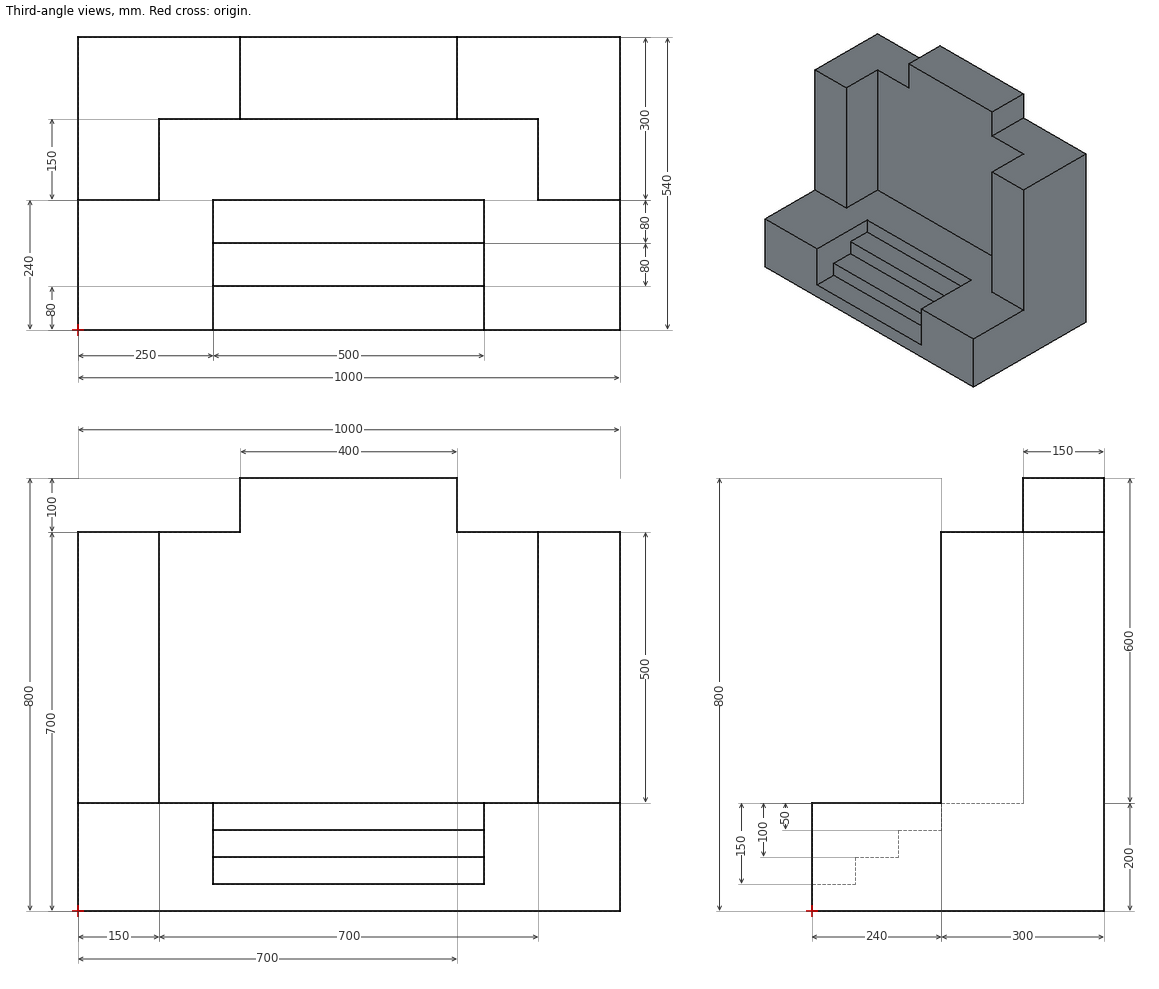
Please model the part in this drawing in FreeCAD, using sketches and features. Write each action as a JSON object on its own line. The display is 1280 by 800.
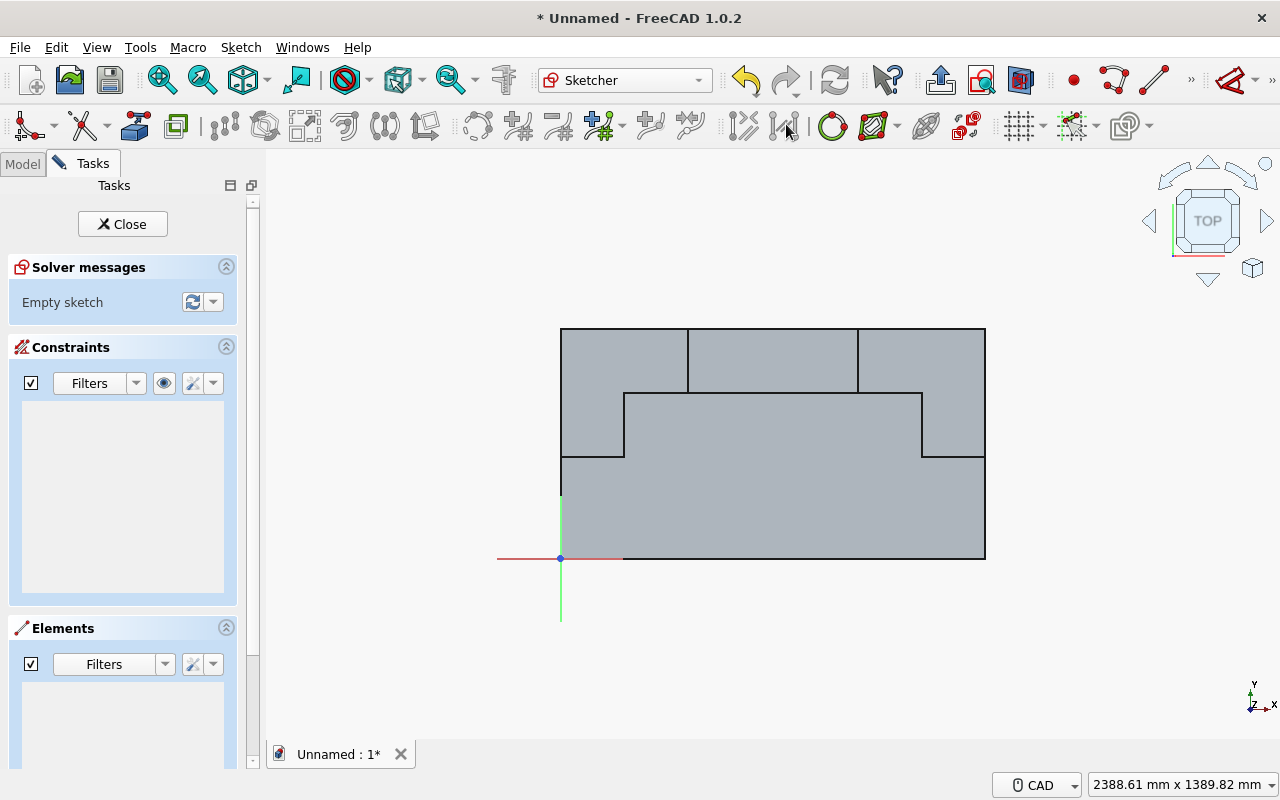
{"action": "scroll", "coordinate": [739, 660], "scroll_direction": "up", "scroll_amount": 3}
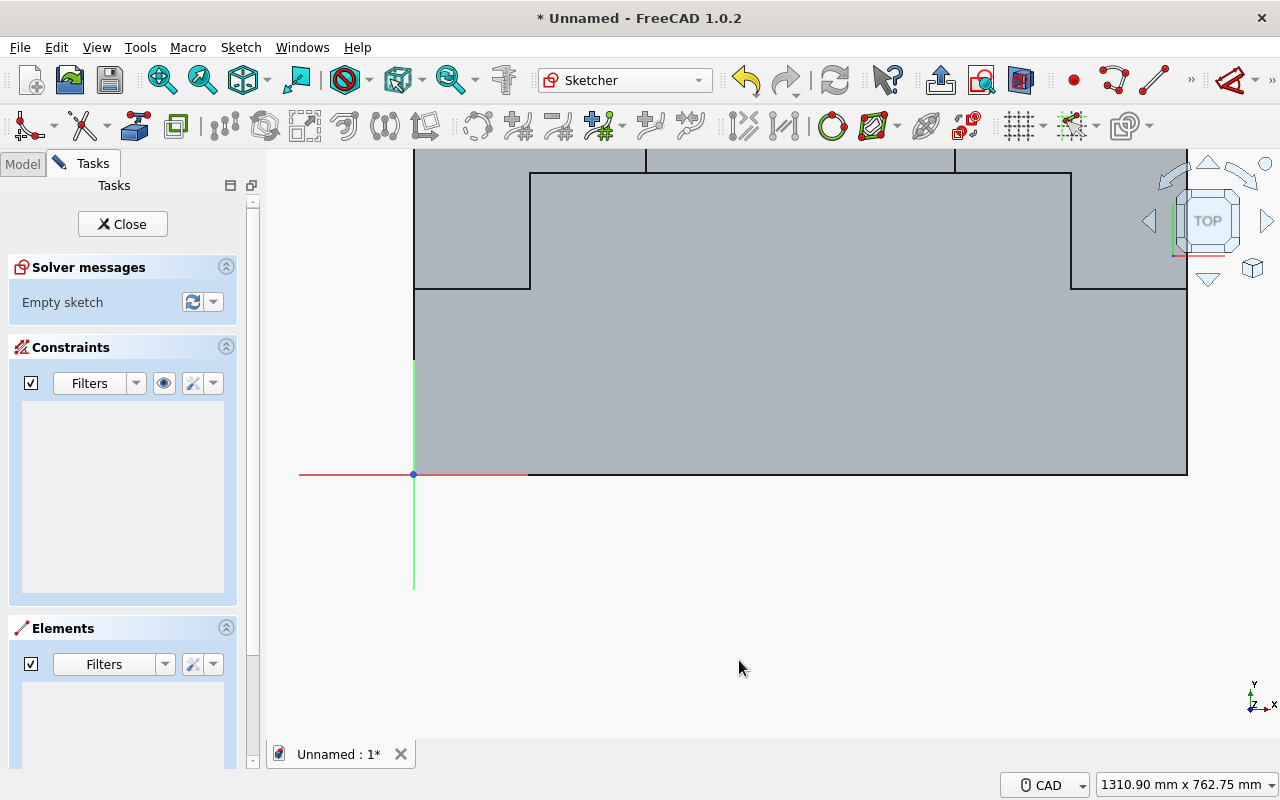
{"action": "key", "text": "g r"}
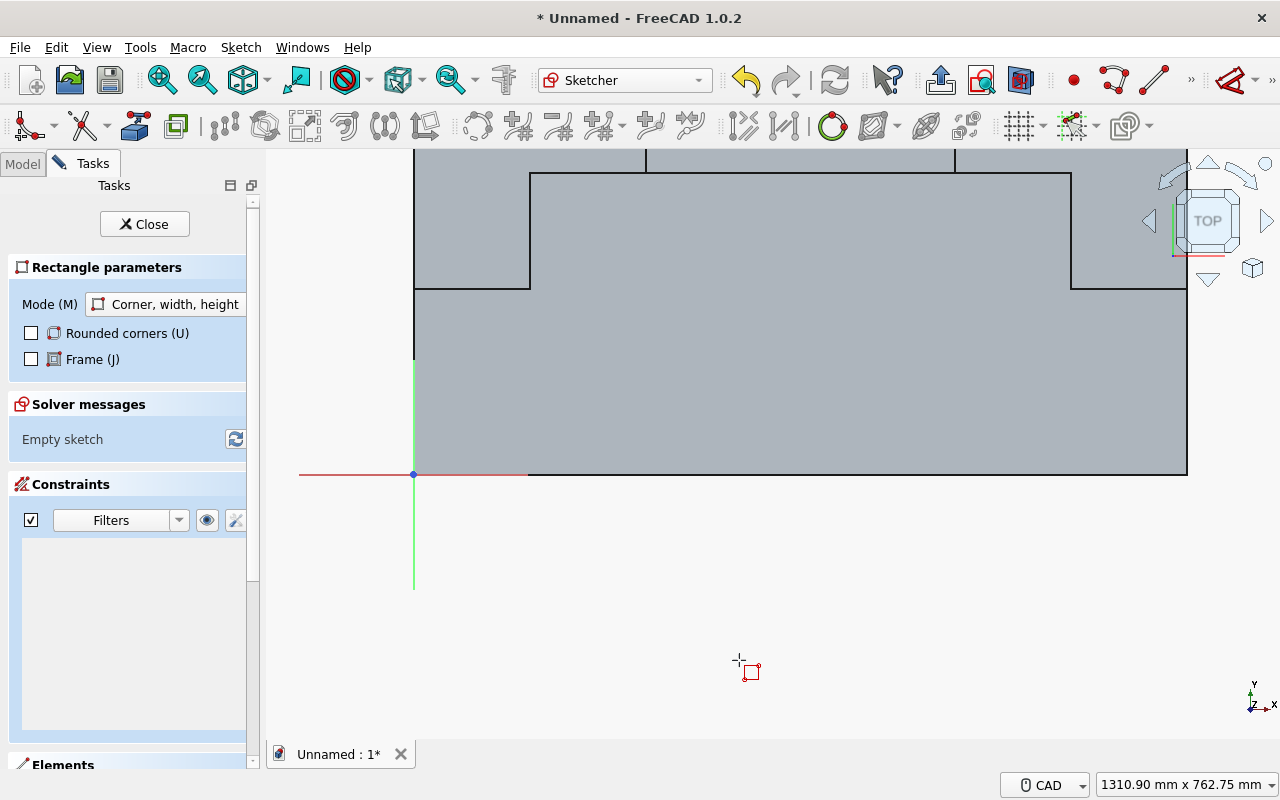
{"action": "left_click", "coordinate": [607, 413]}
{"action": "left_click", "coordinate": [994, 475]}
{"action": "key", "text": "Escape"}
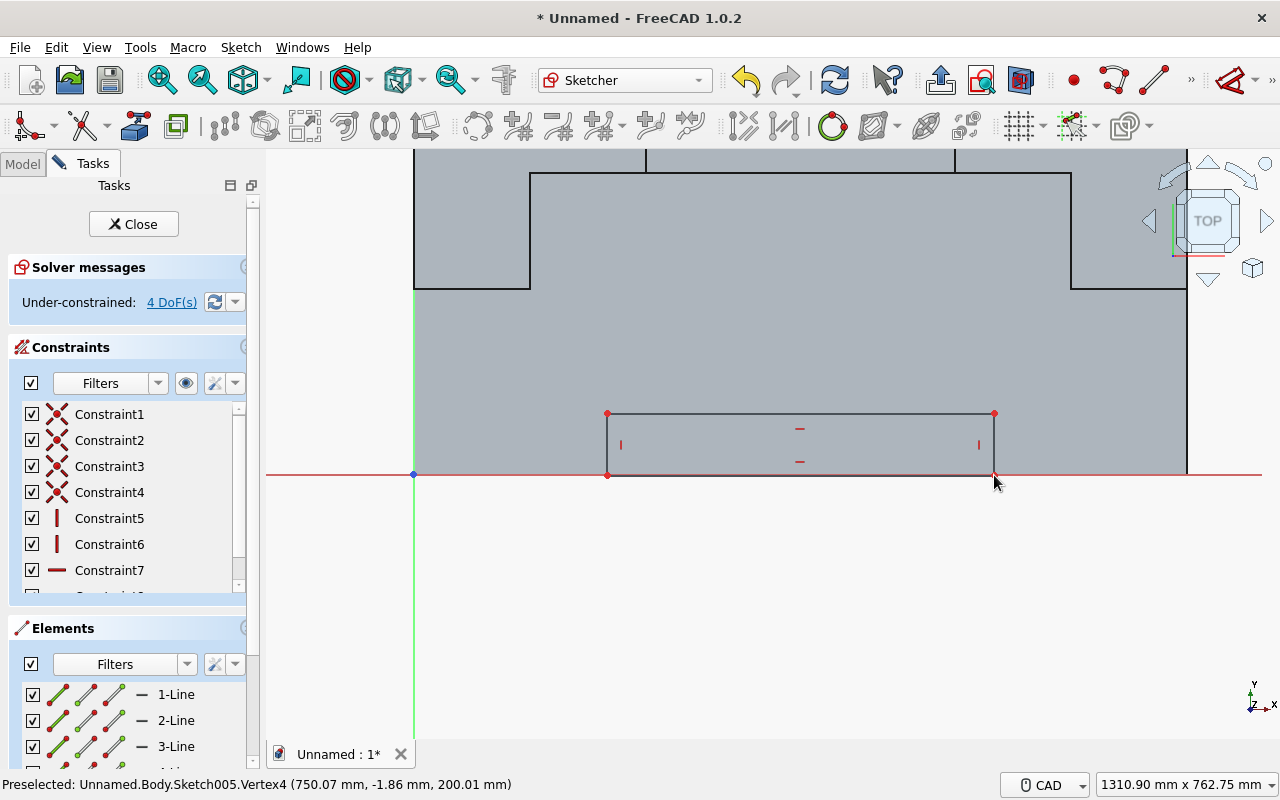
{"action": "left_click", "coordinate": [607, 476]}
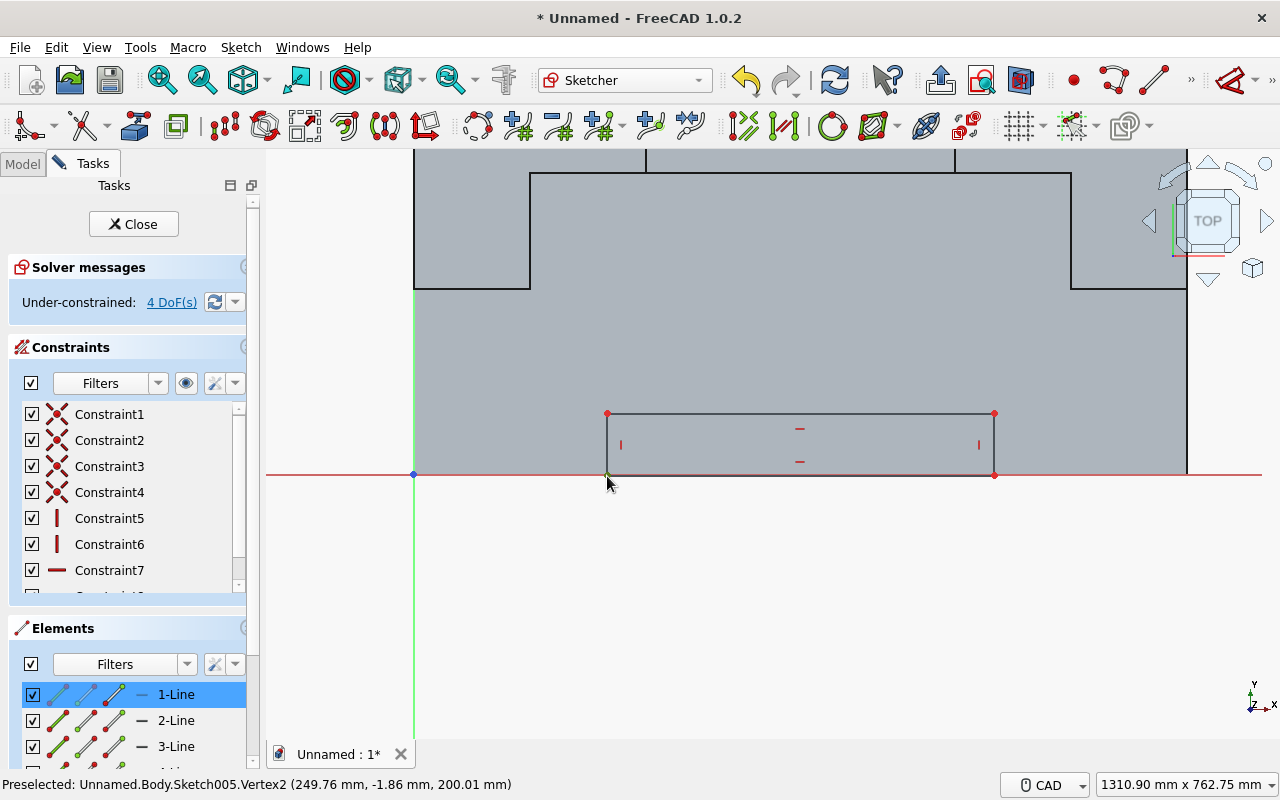
{"action": "left_click", "coordinate": [353, 475]}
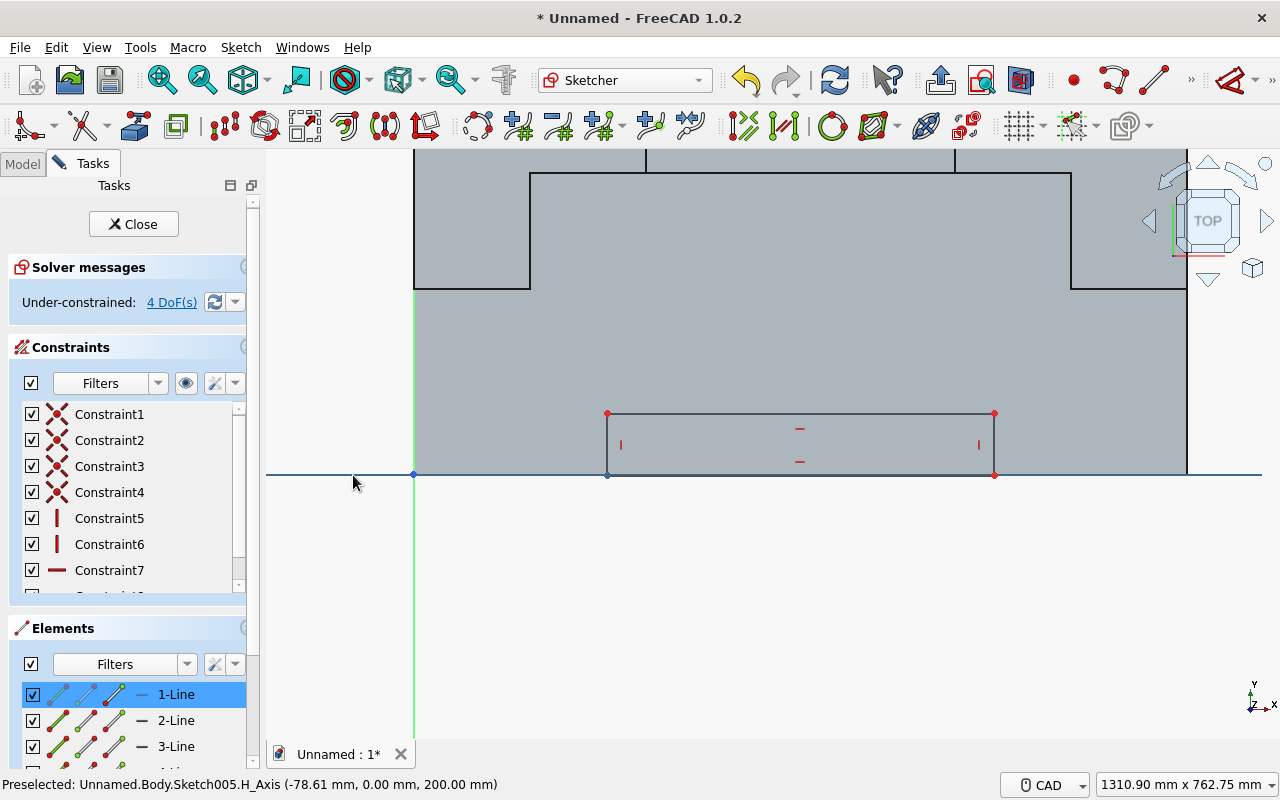
{"action": "key", "text": "c"}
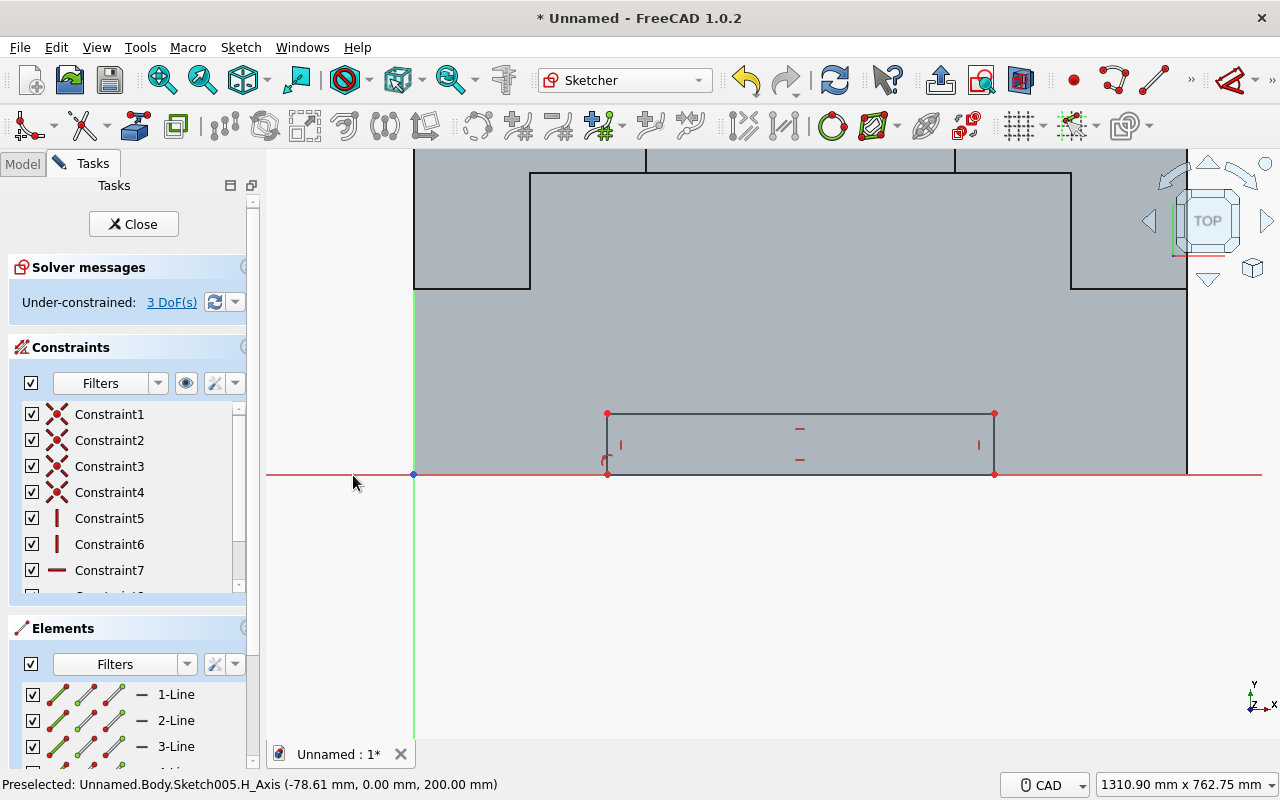
{"action": "left_click", "coordinate": [1230, 80]}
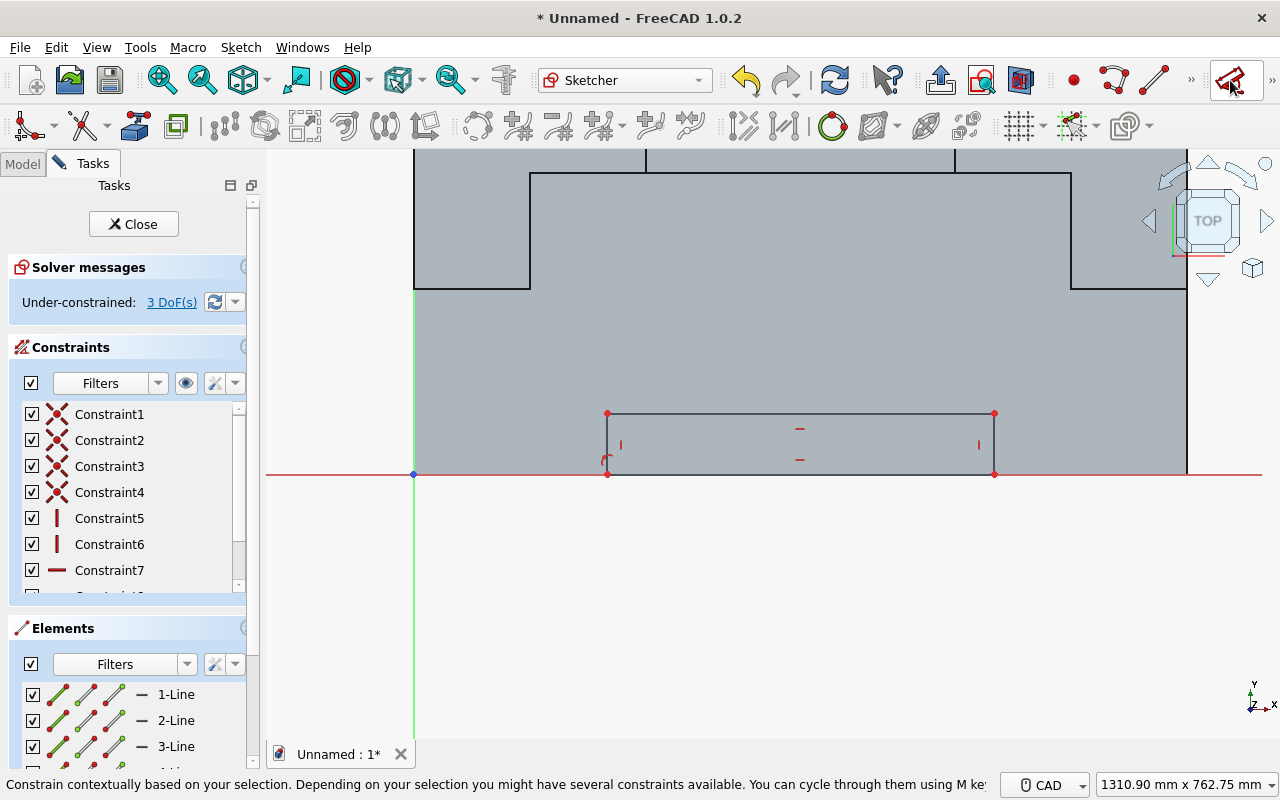
{"action": "left_click", "coordinate": [607, 432]}
{"action": "left_click", "coordinate": [573, 444]}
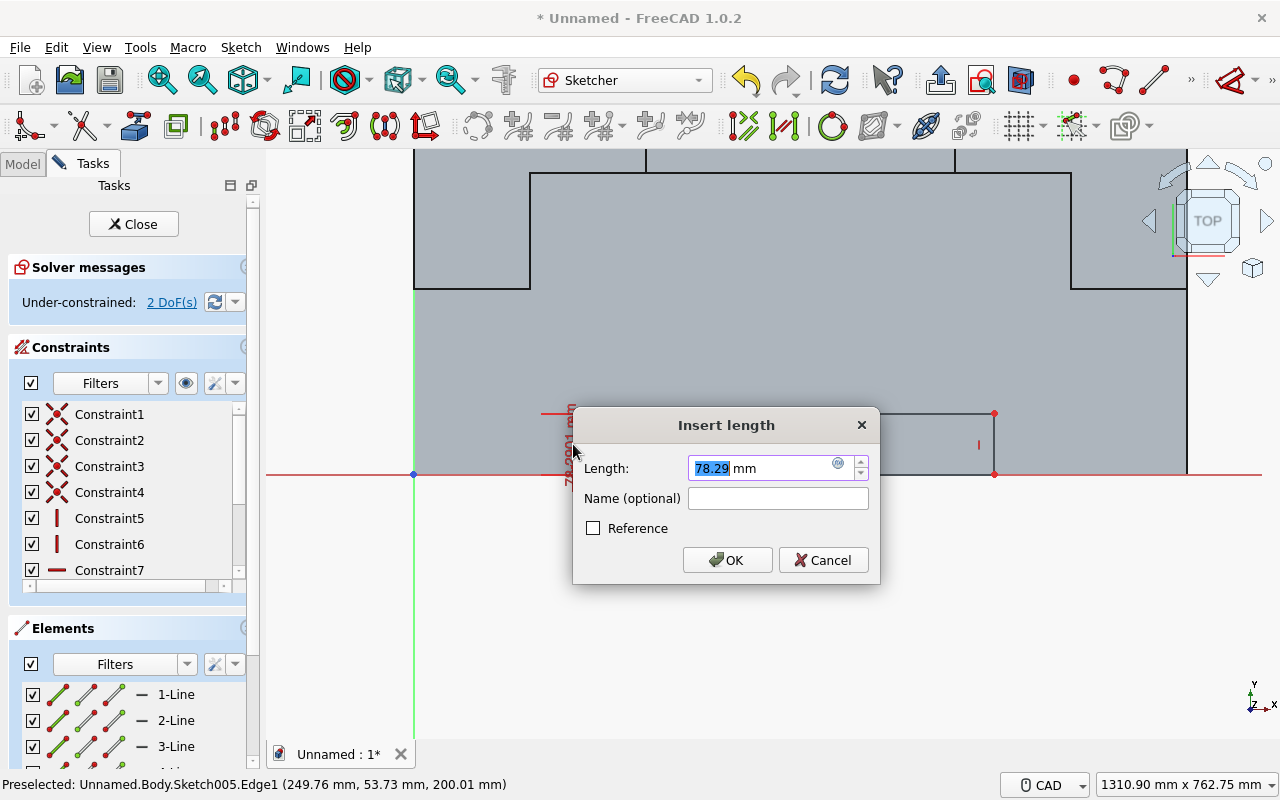
{"action": "type", "text": "80"}
{"action": "key", "text": "Return"}